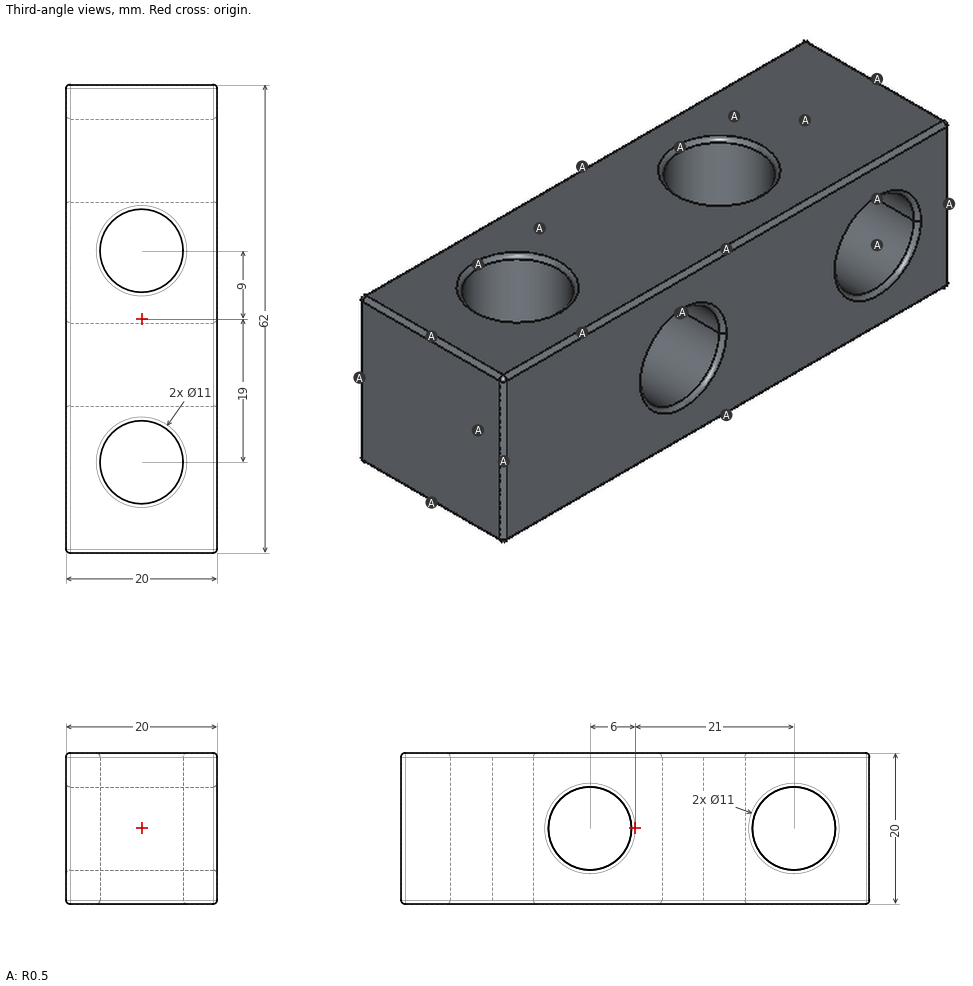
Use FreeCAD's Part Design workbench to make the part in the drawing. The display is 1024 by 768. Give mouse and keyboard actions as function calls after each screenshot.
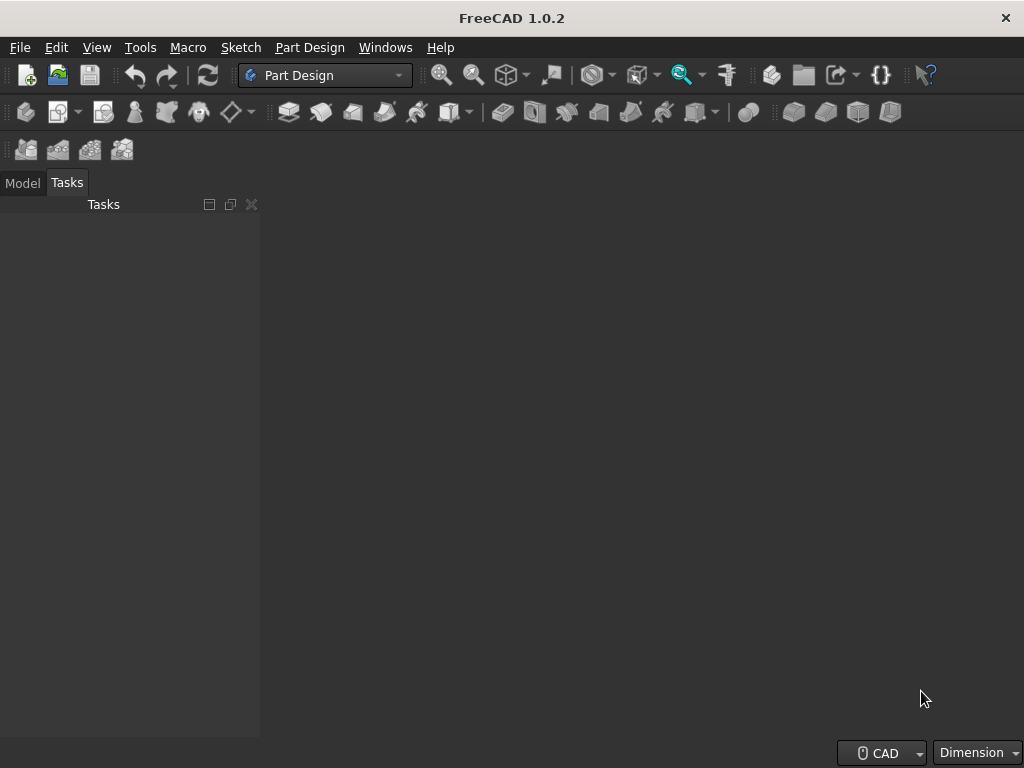
key(ctrl+n)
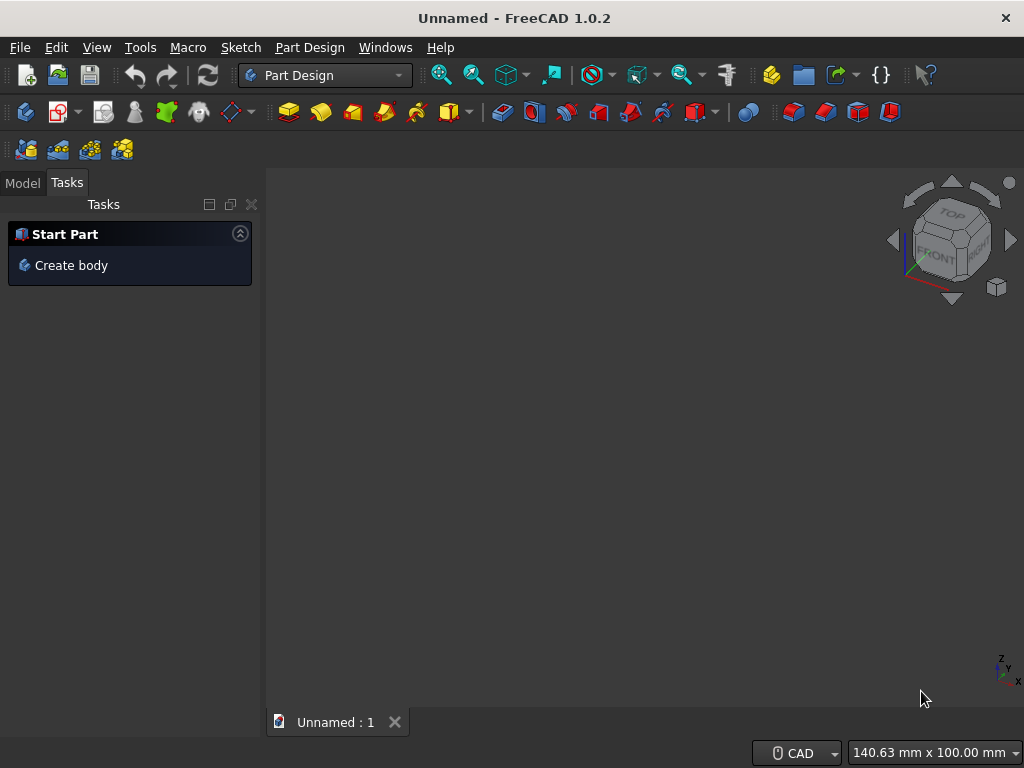
click(58, 112)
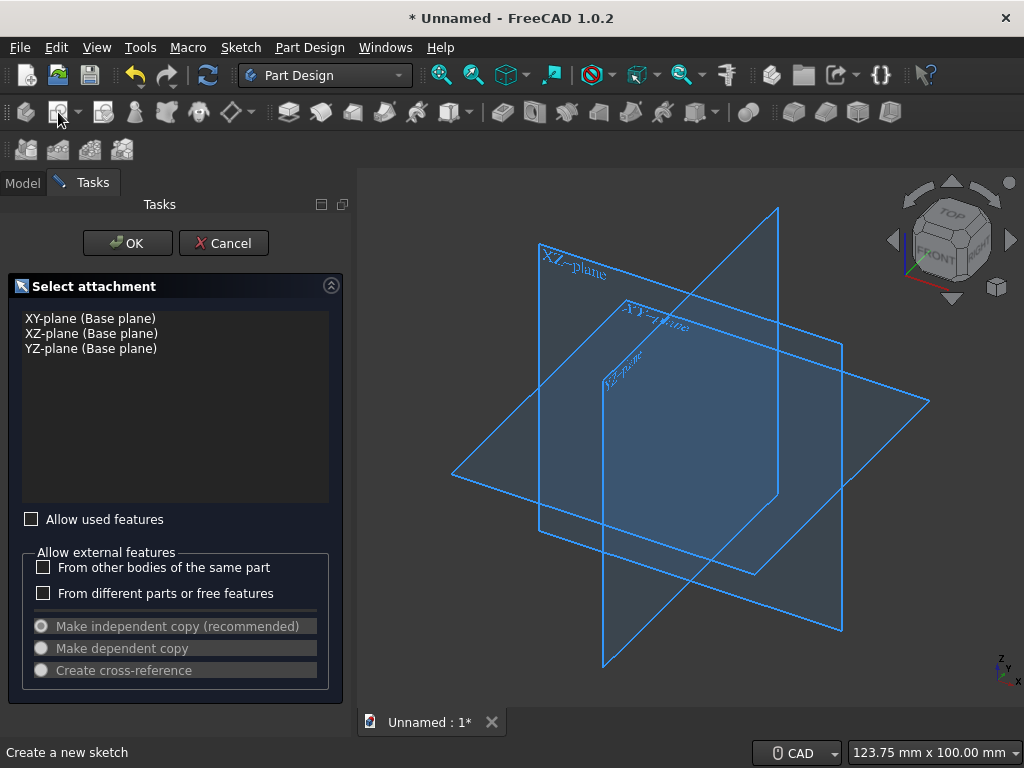
click(82, 318)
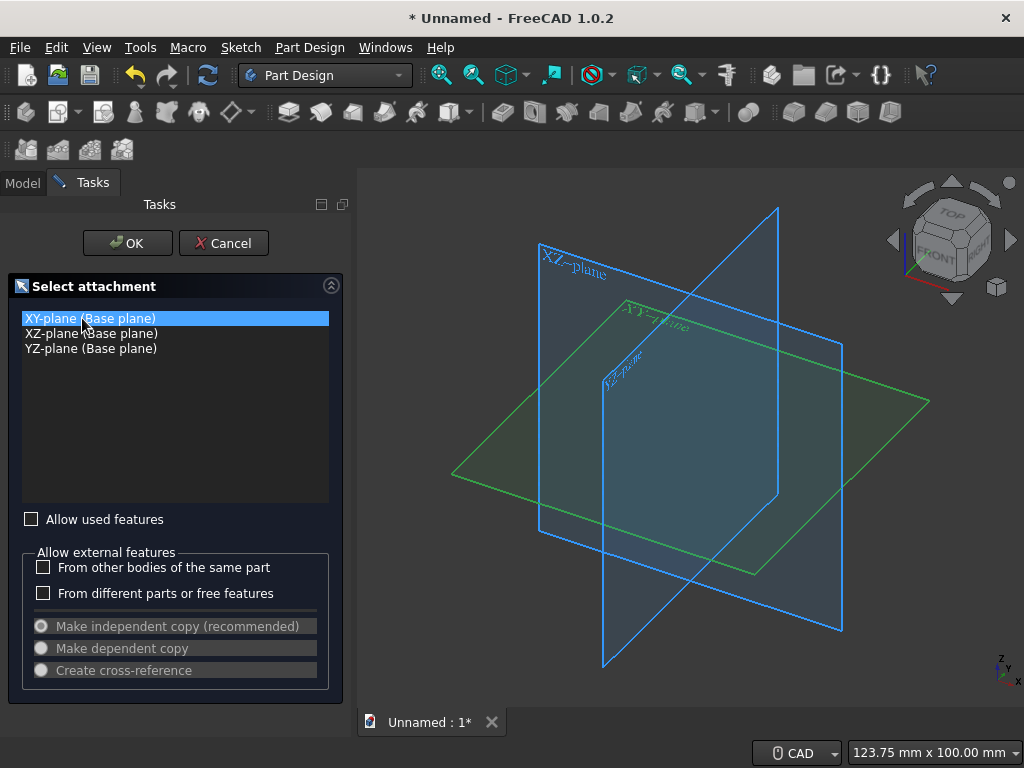
click(128, 243)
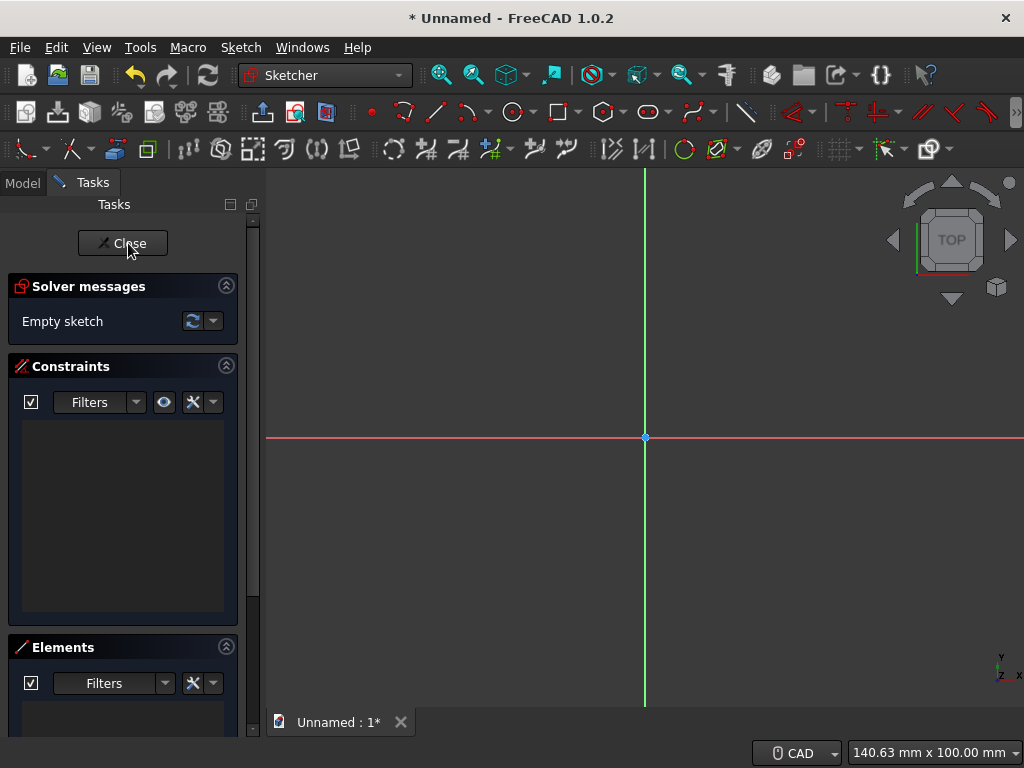
click(580, 112)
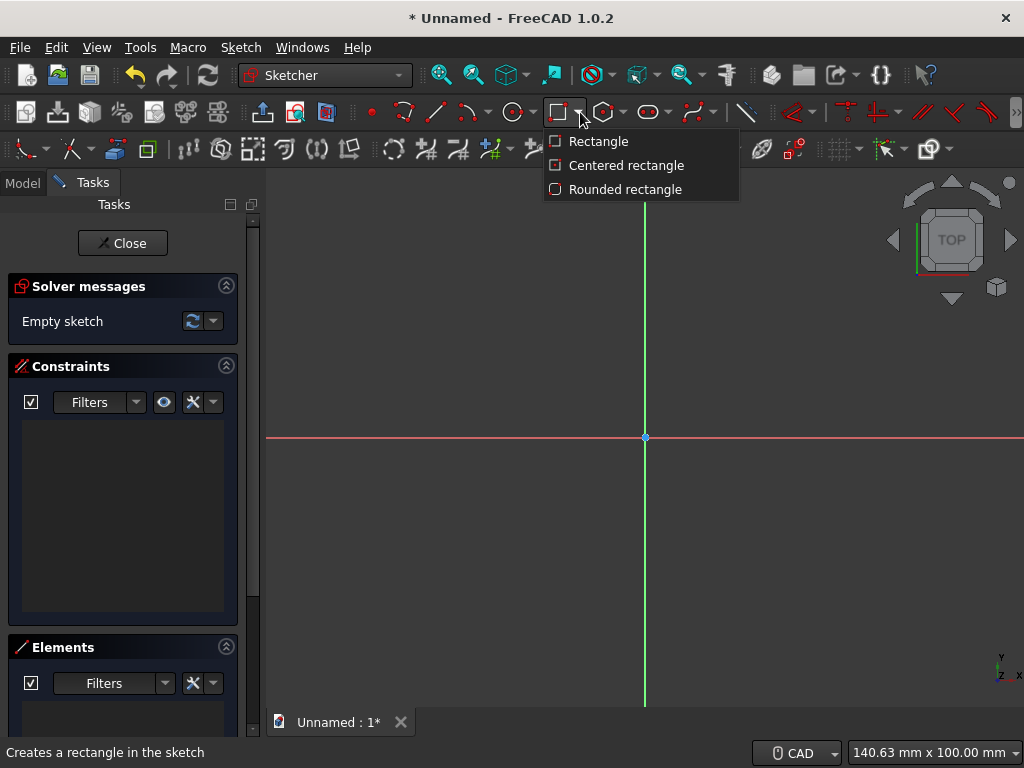
click(642, 165)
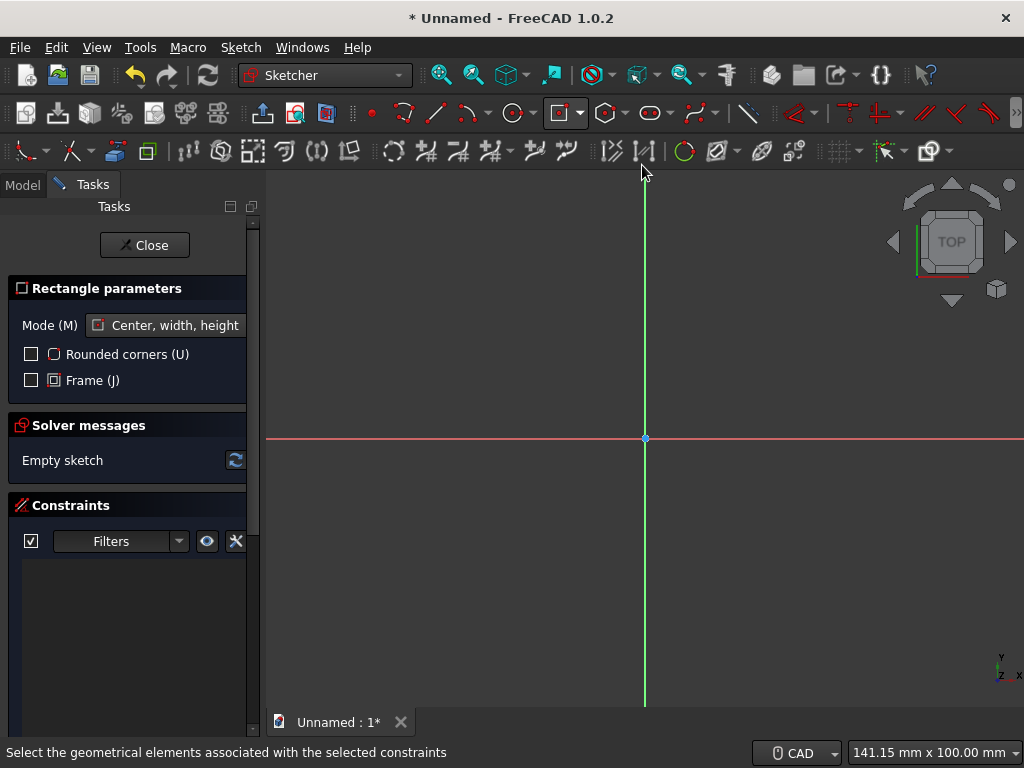
click(645, 438)
move(699, 272)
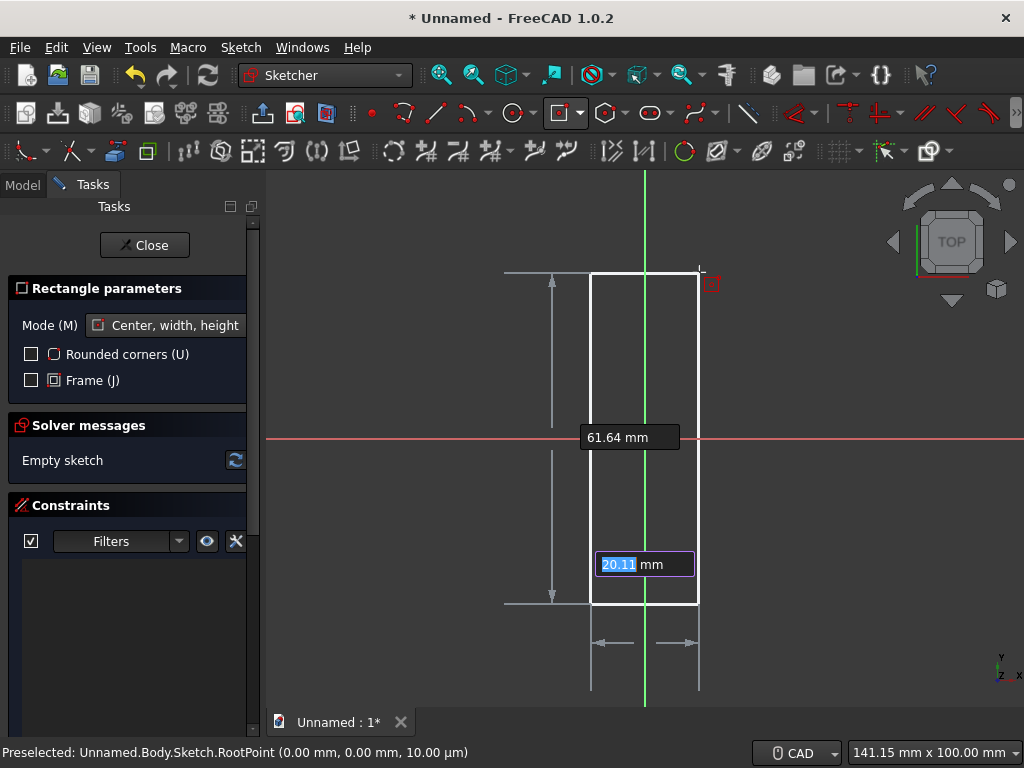
text(20)
key(Tab)
text(62)
key(Return)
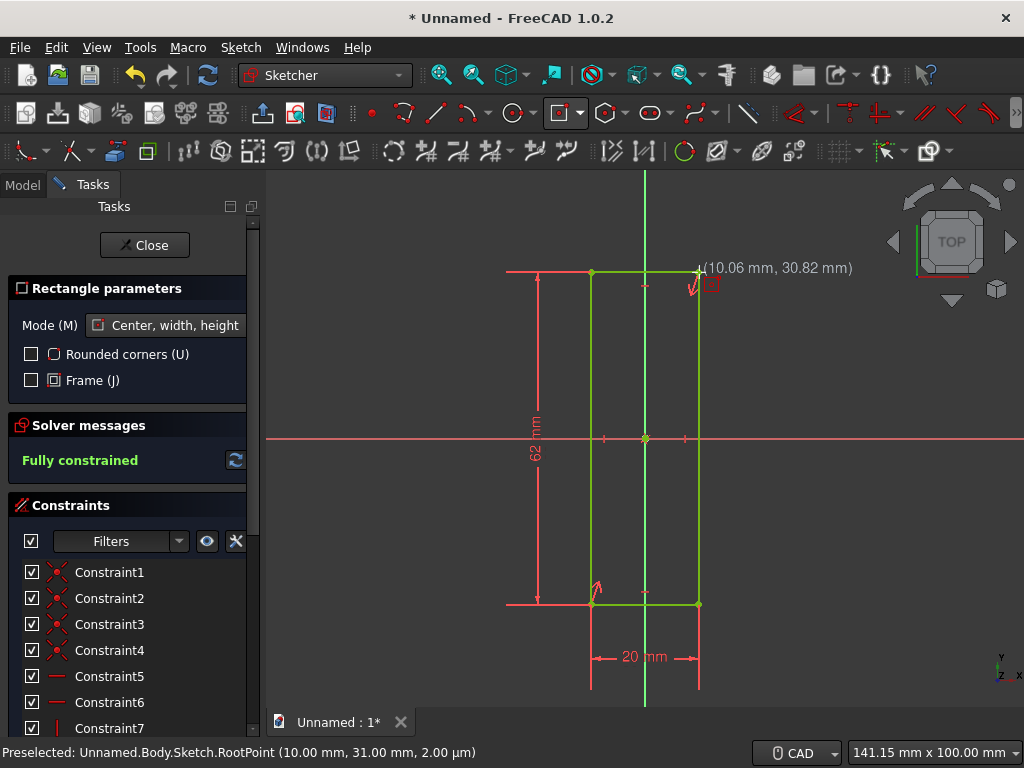
key(g)
key(c)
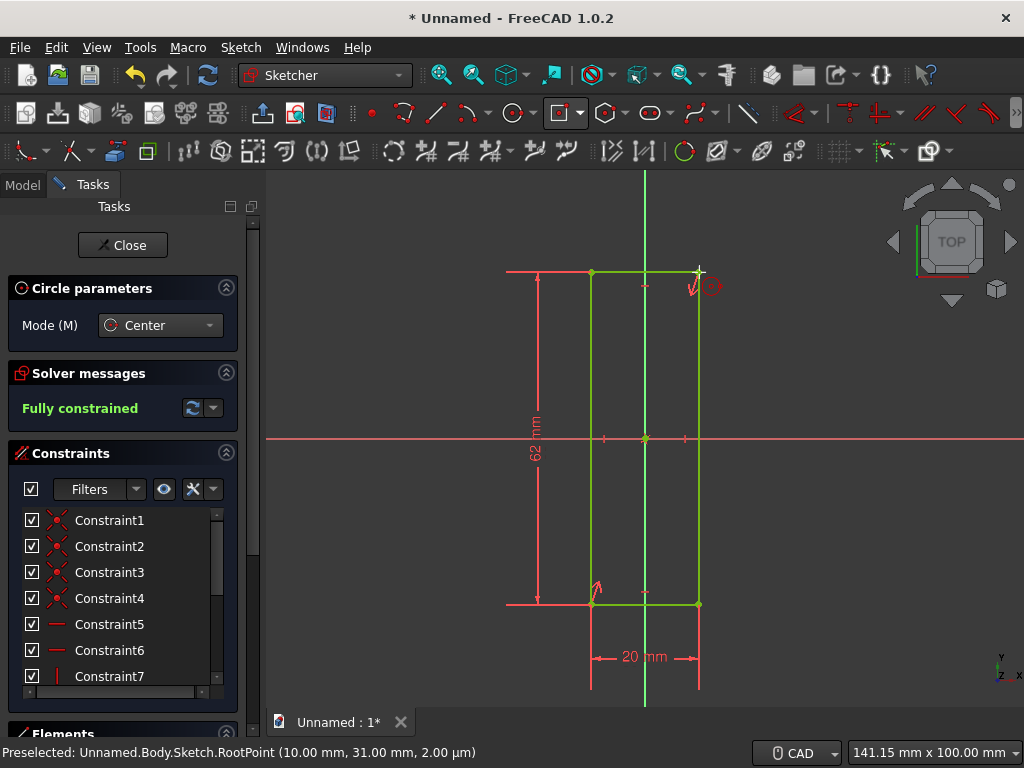
click(645, 541)
move(666, 520)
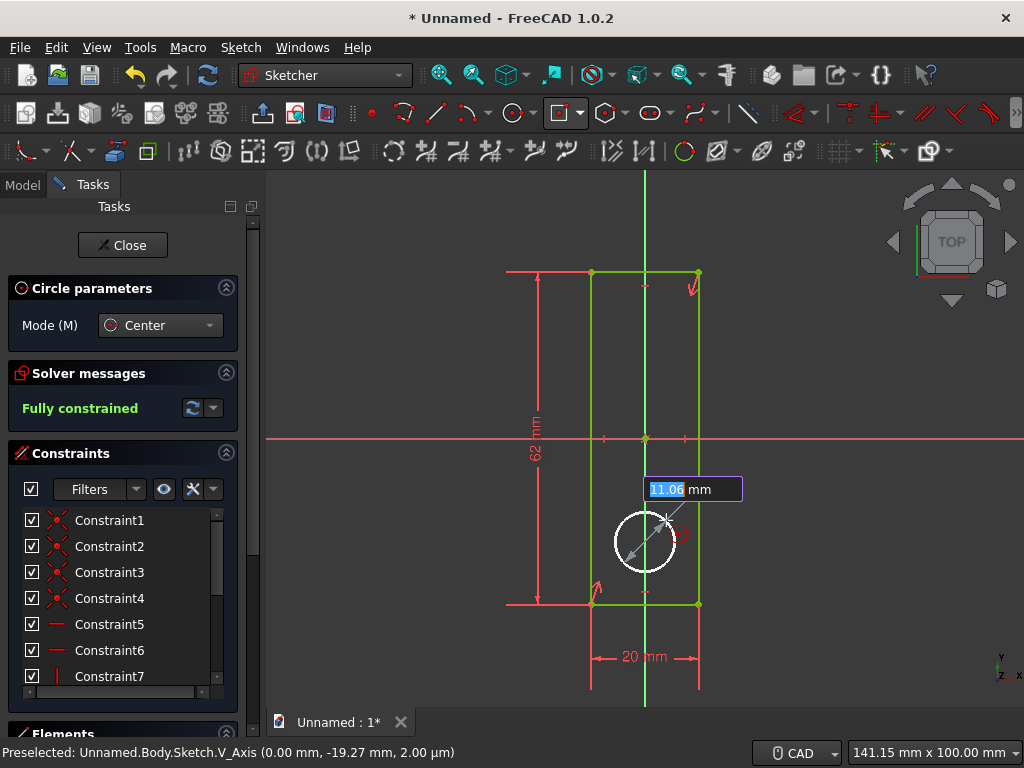
text(11)
key(Return)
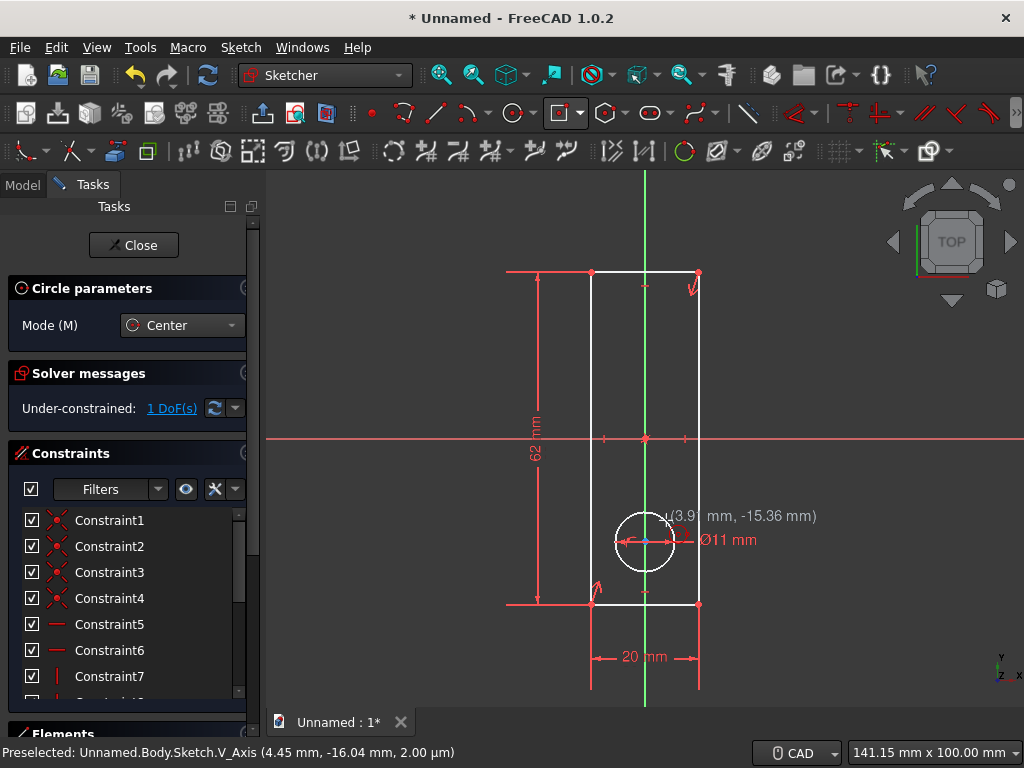
click(645, 390)
move(666, 369)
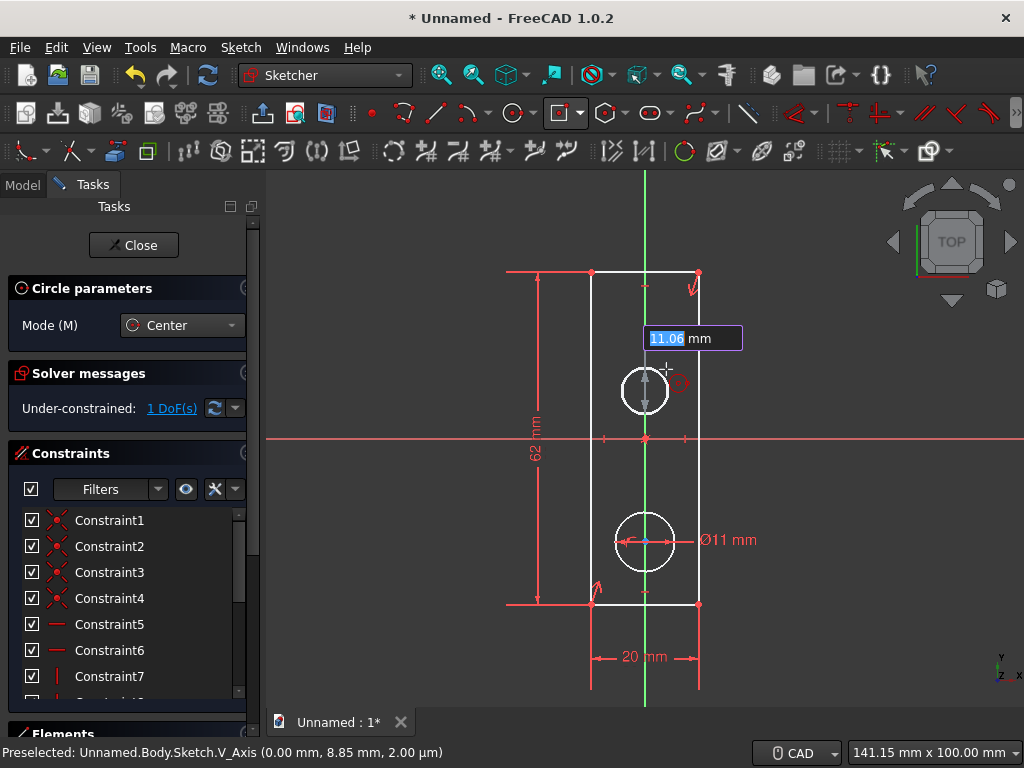
text(11)
key(Return)
key(Escape)